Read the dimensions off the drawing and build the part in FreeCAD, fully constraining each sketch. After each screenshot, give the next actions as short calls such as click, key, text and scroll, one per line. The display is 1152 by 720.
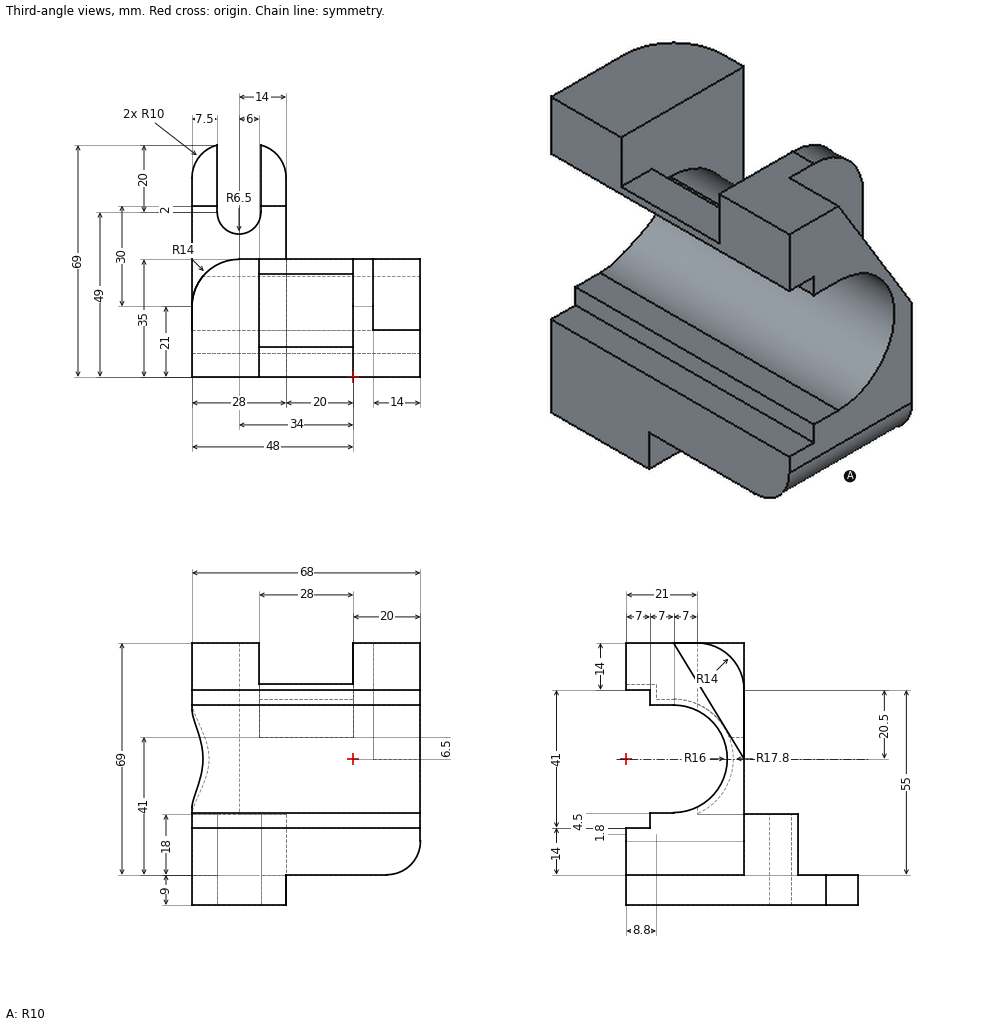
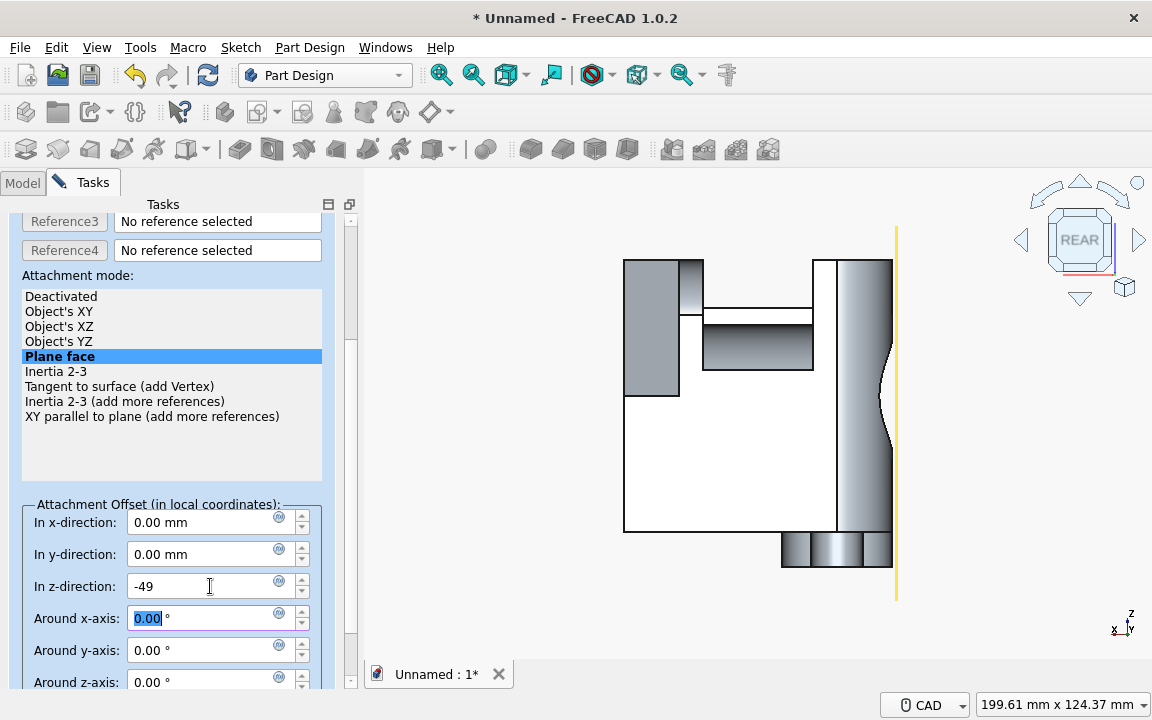
scroll(351, 451, up, 4)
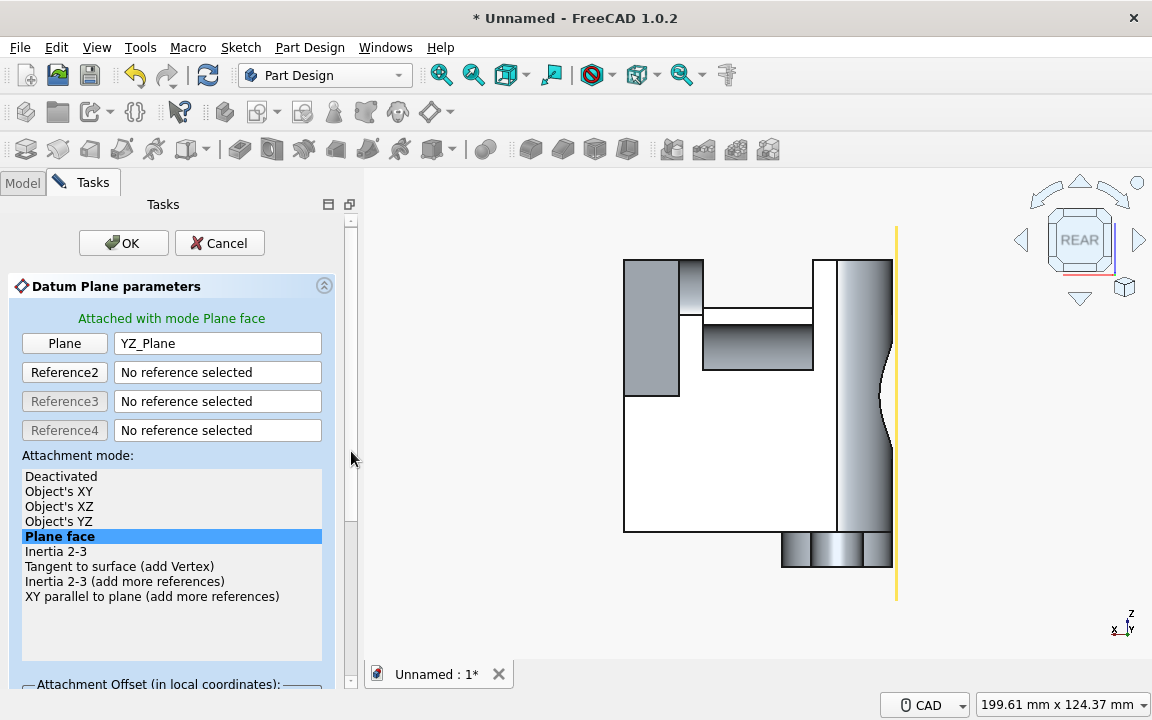
click(124, 243)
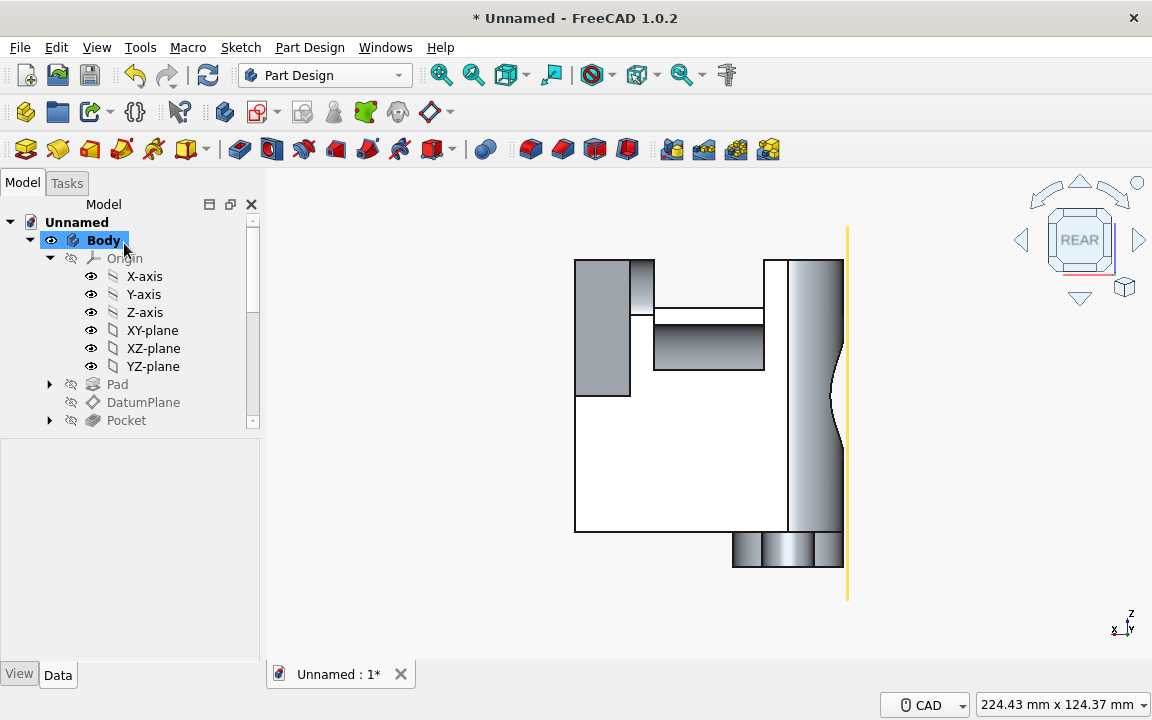
scroll(100, 326, down, 3)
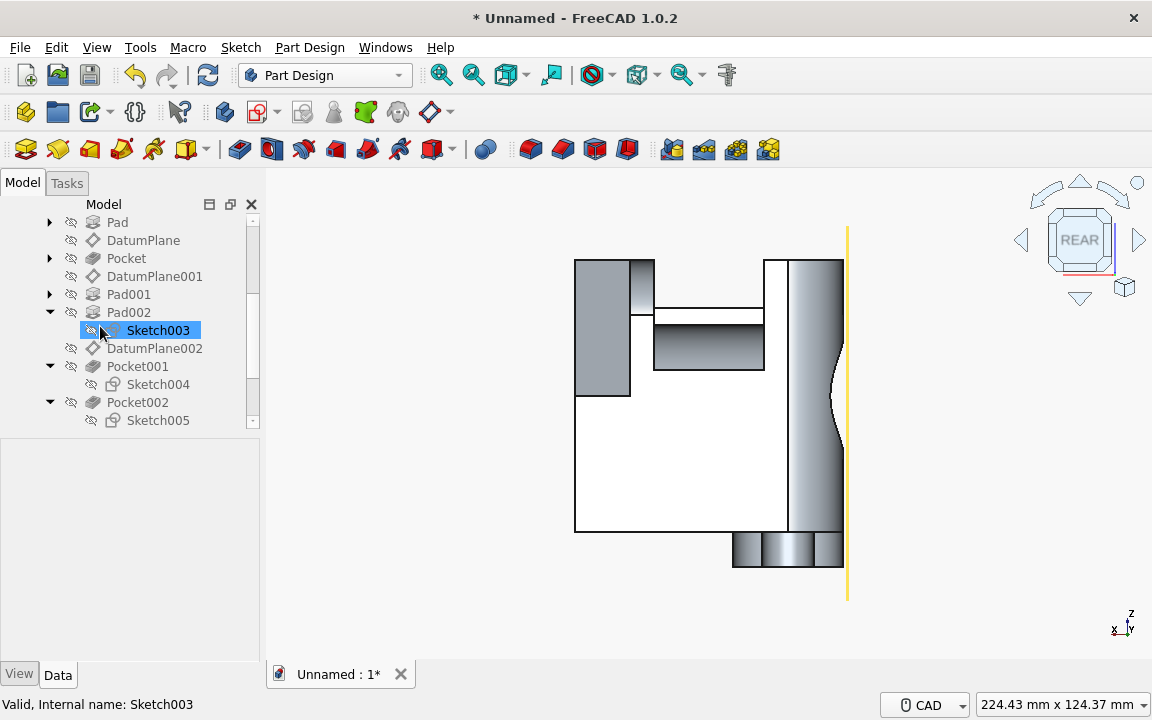
scroll(140, 326, up, 15)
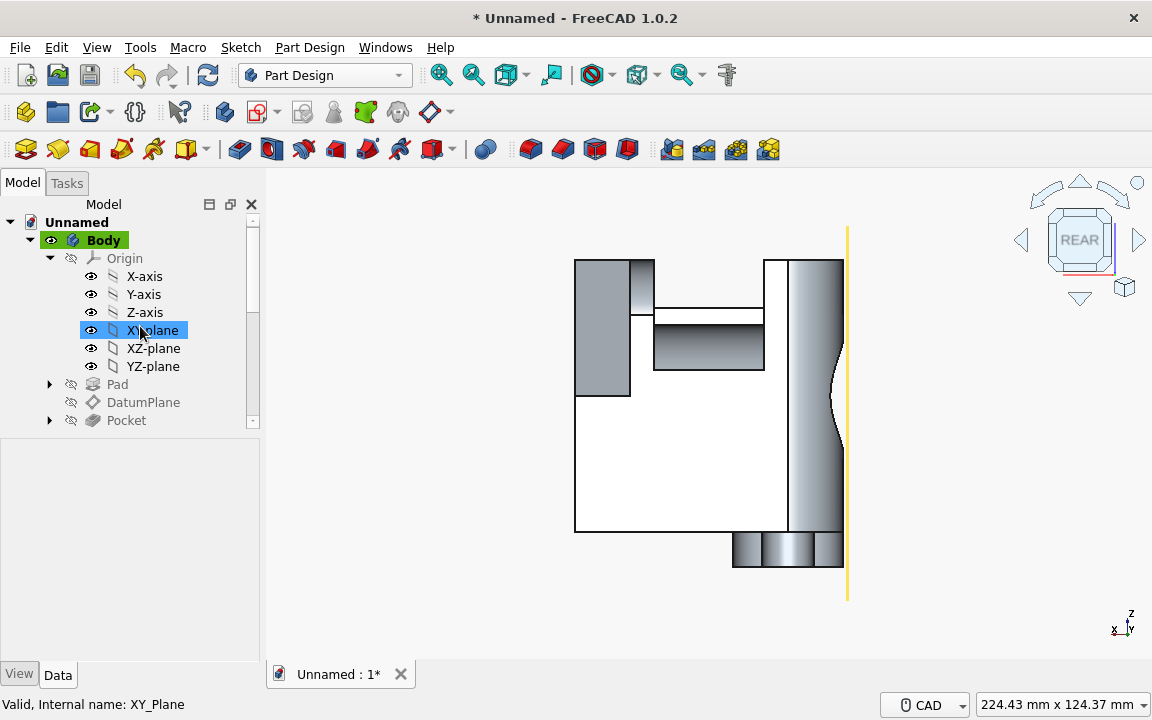
scroll(100, 326, down, 6)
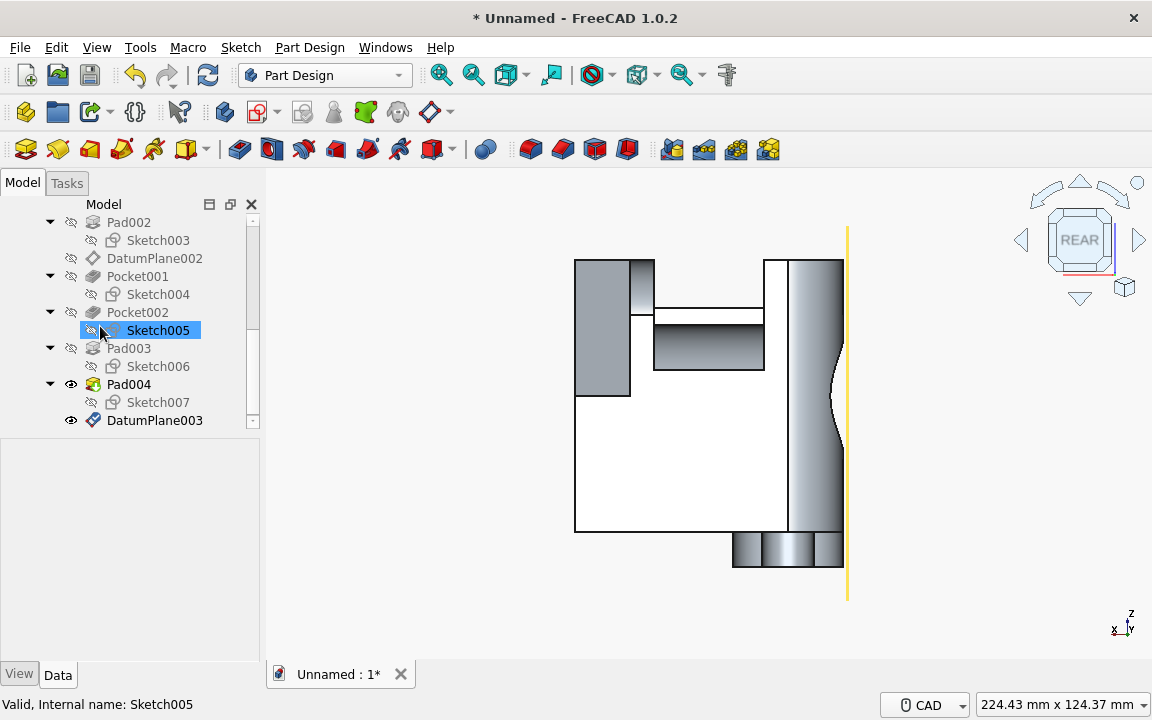
click(116, 420)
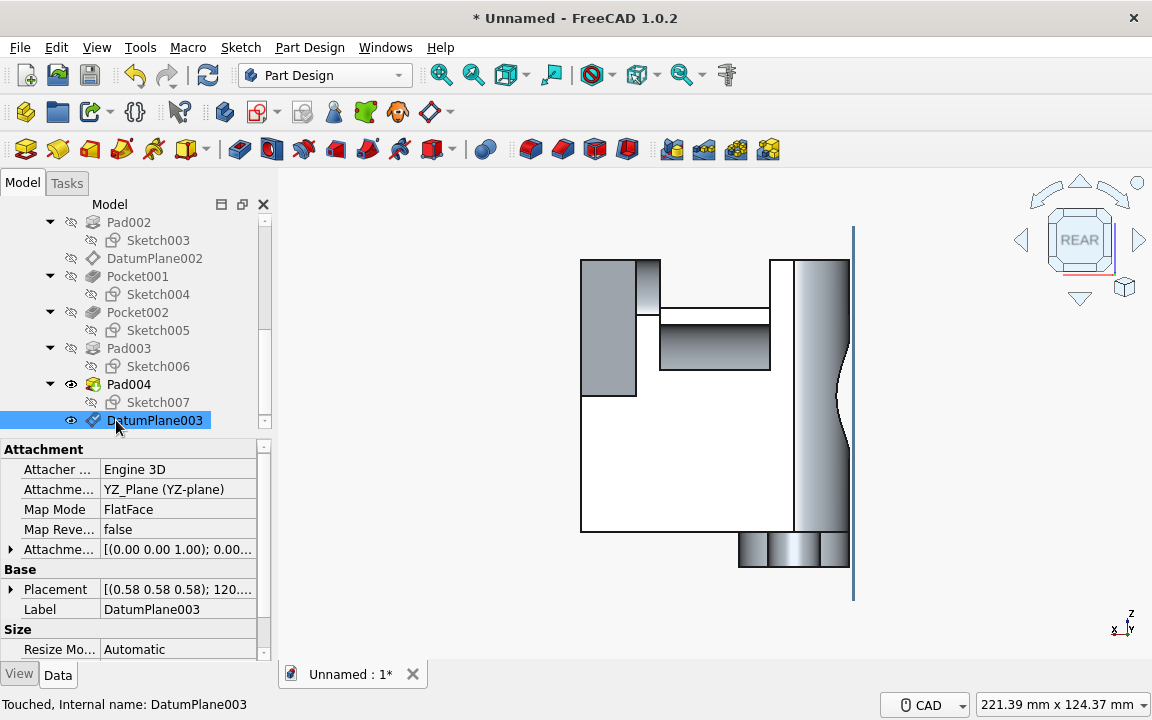
click(258, 112)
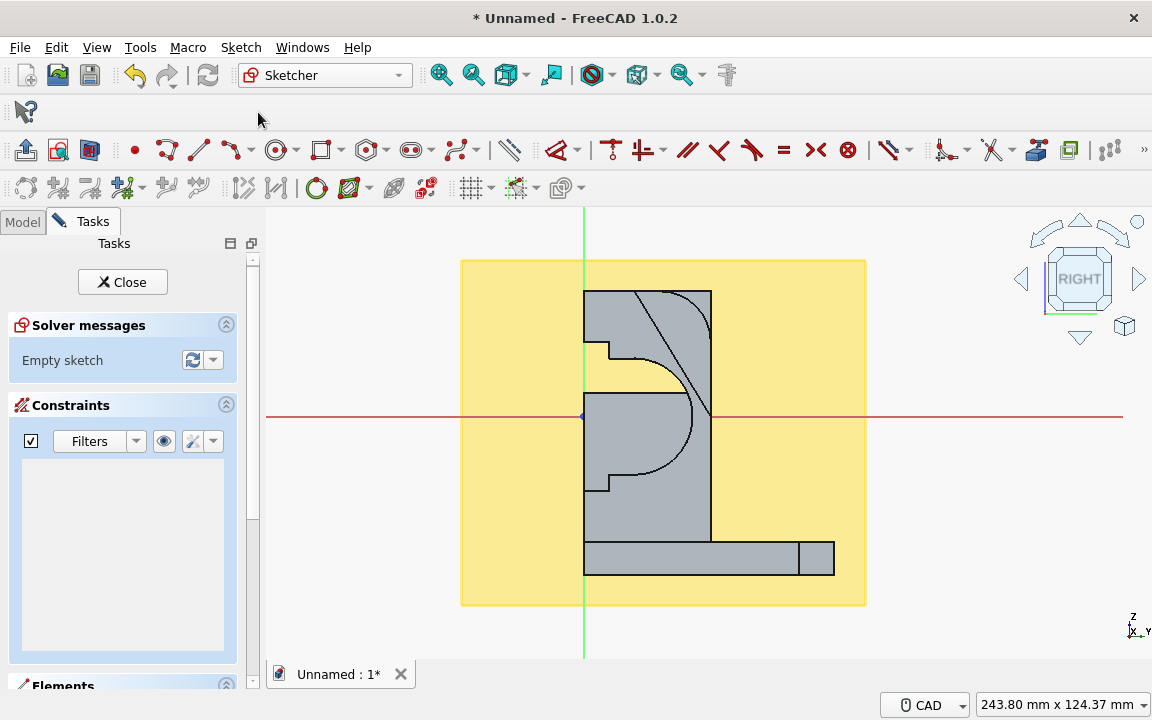
click(90, 150)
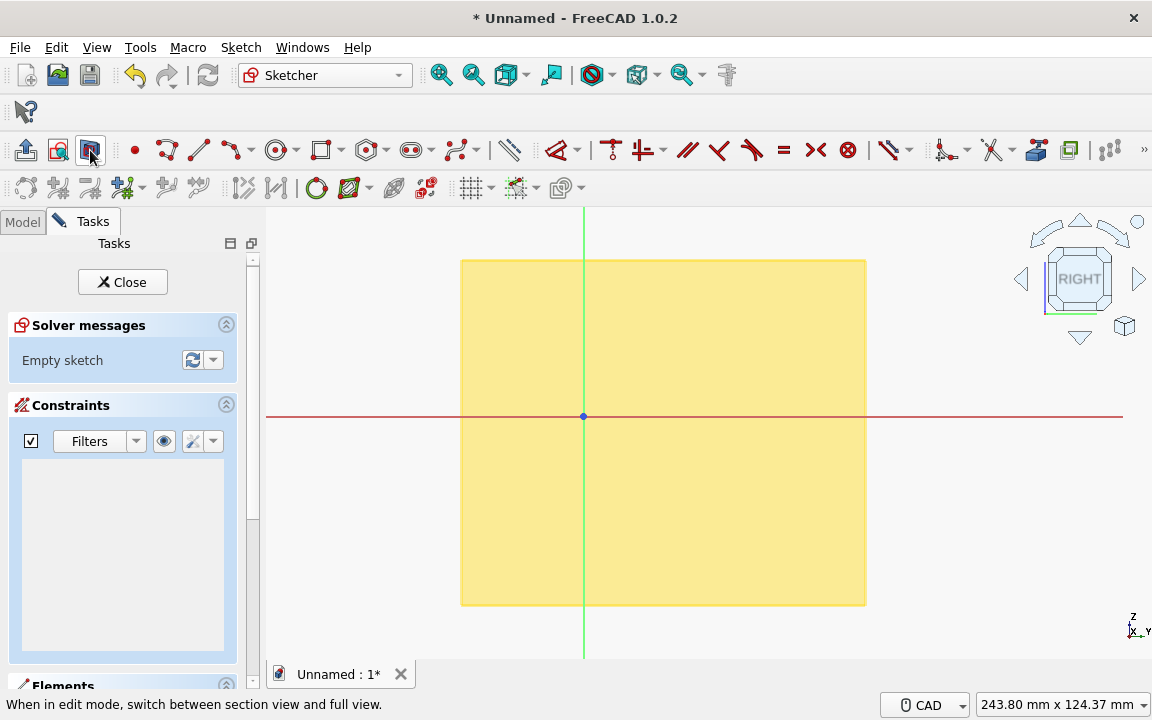
scroll(635, 397, up, 3)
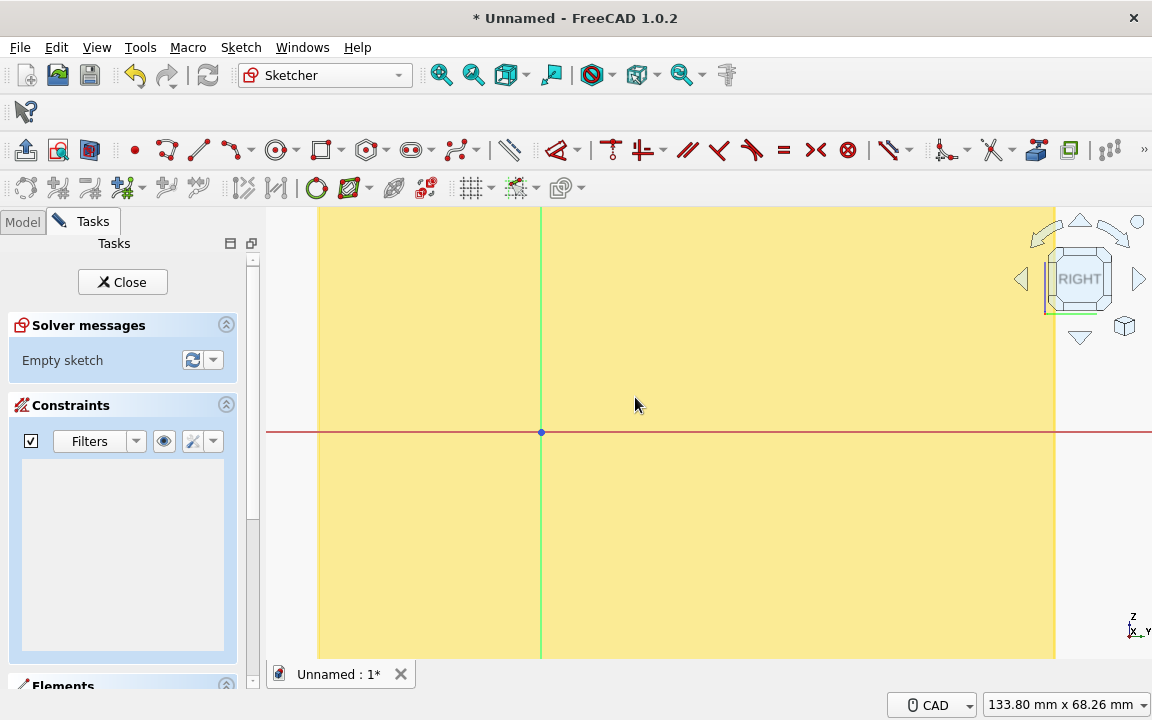
key(g)
key(m)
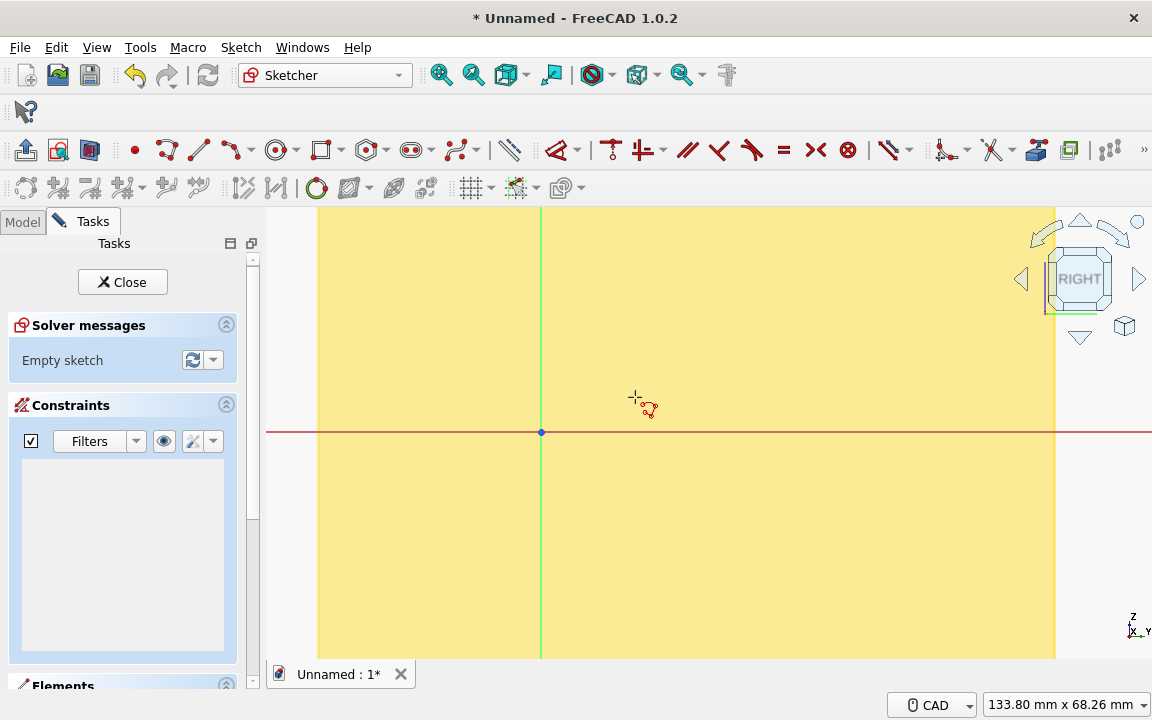
click(634, 327)
click(587, 327)
click(587, 297)
click(541, 297)
click(550, 568)
click(587, 568)
click(587, 538)
click(634, 538)
right_click(634, 538)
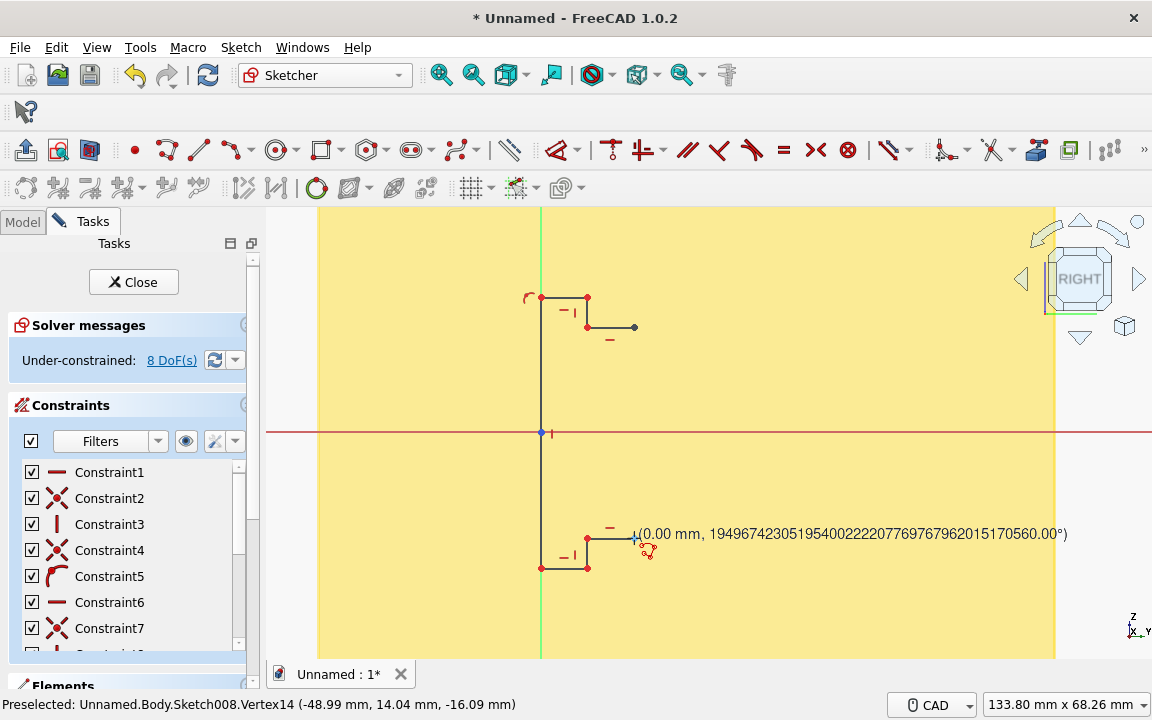
click(232, 150)